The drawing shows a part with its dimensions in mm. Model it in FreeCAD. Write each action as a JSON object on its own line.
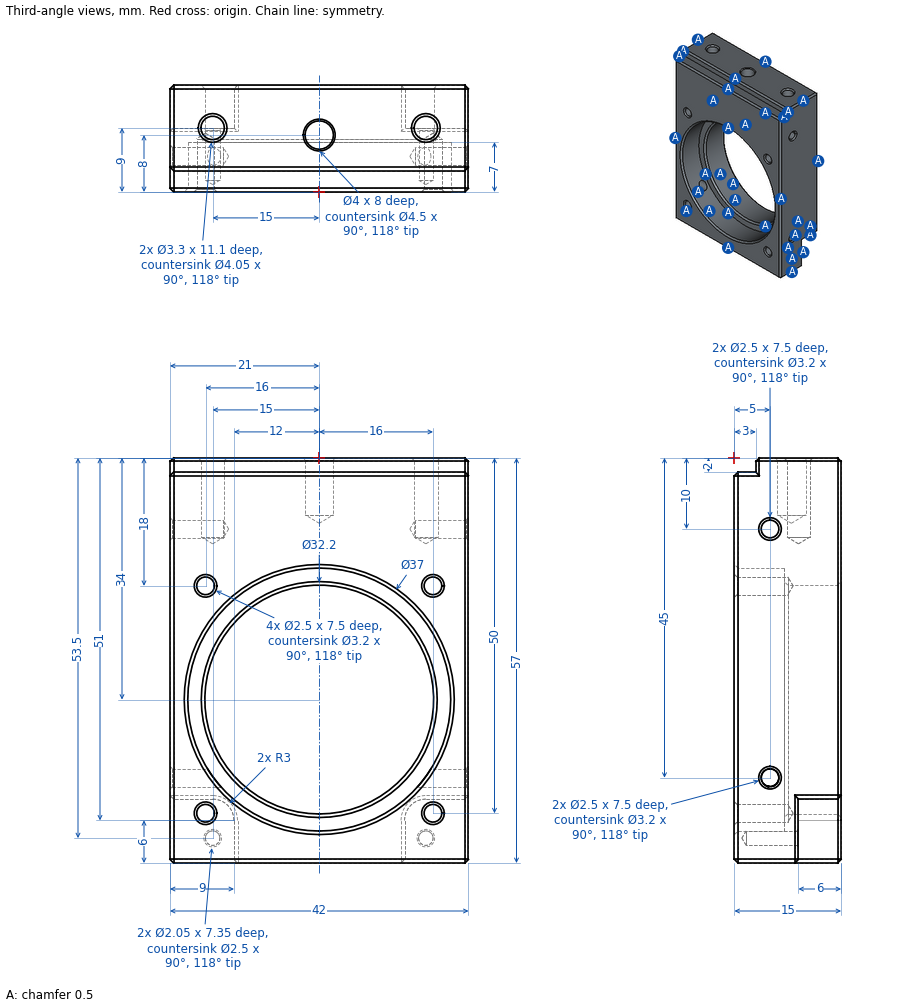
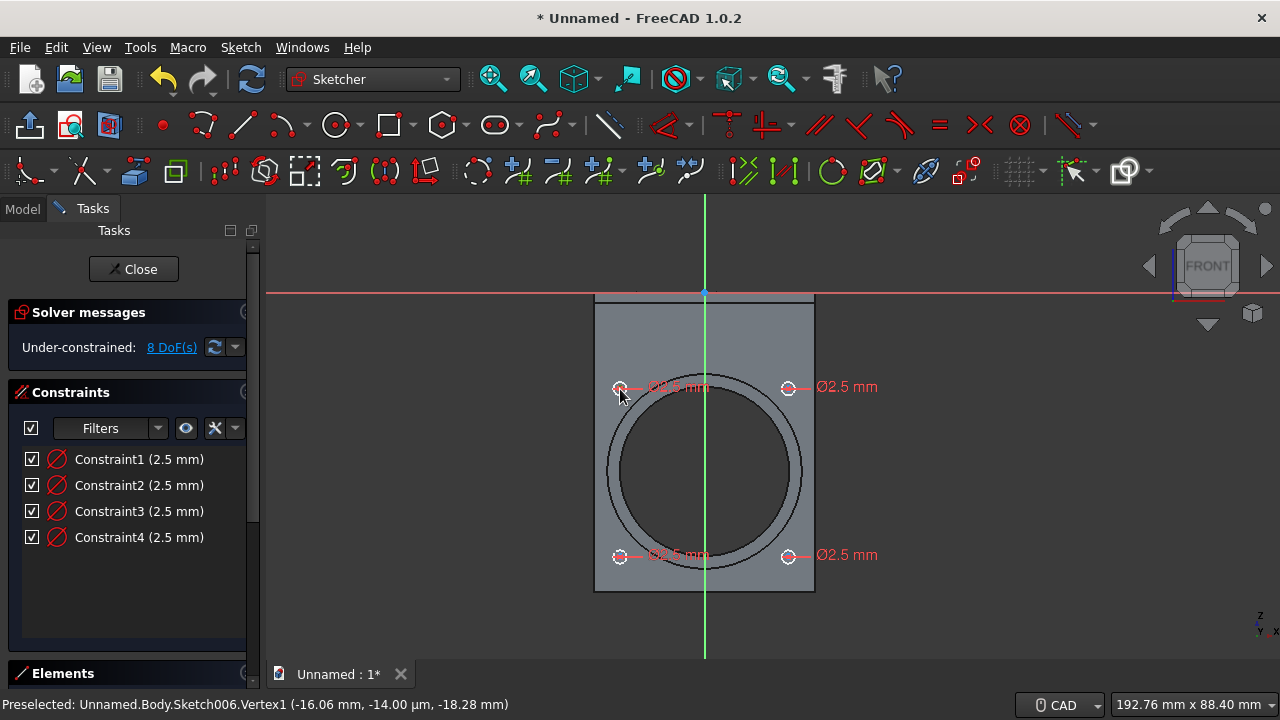
{"action": "left_click", "coordinate": [788, 389]}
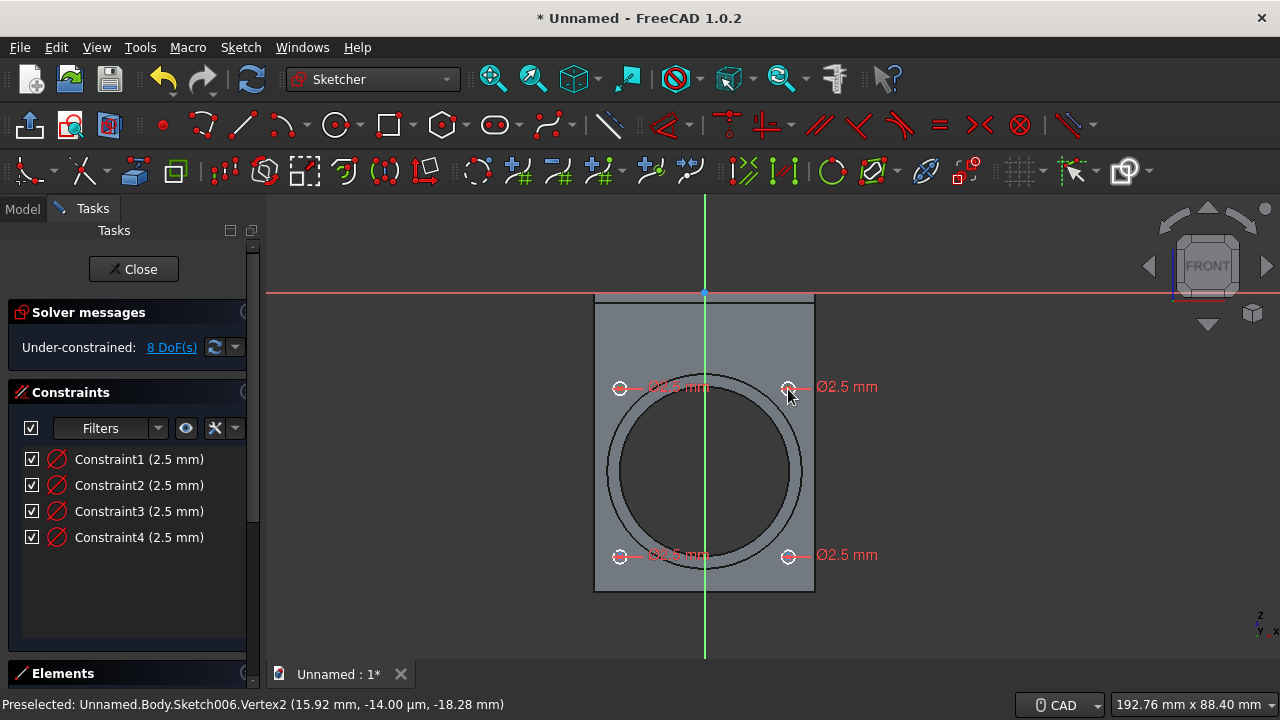
{"action": "left_click", "coordinate": [705, 602]}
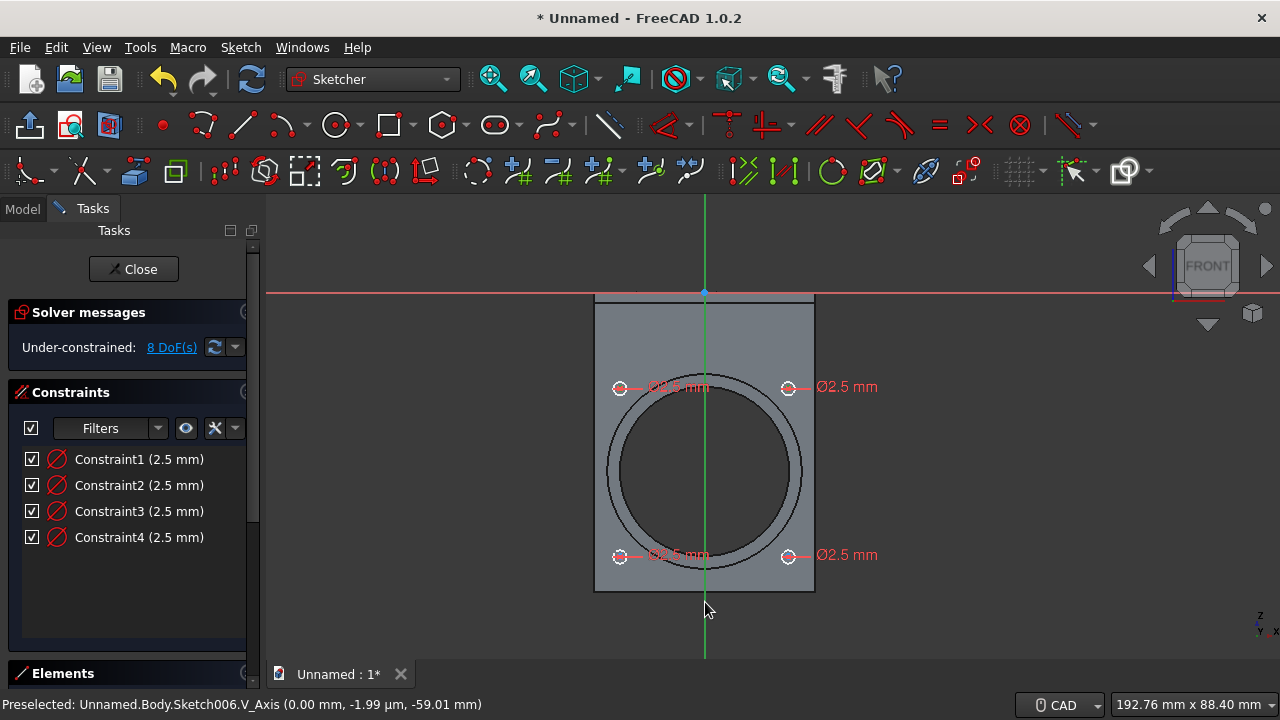
{"action": "key", "text": "s"}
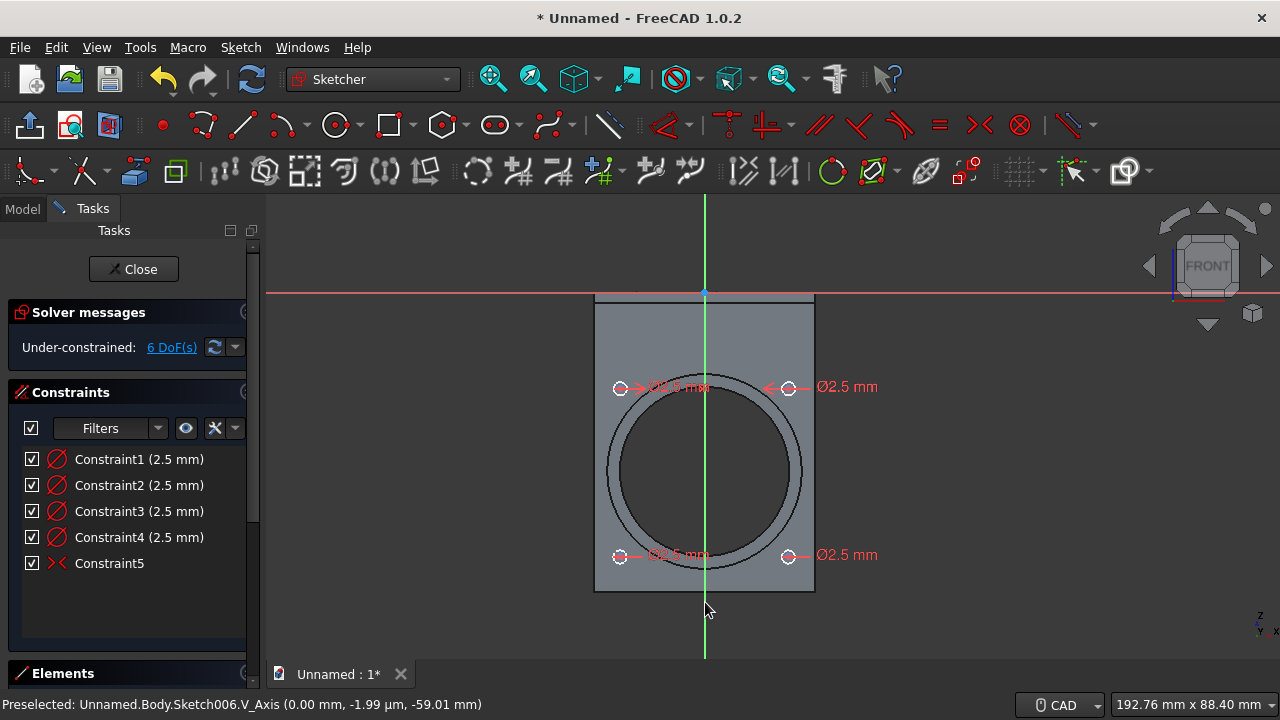
{"action": "left_click", "coordinate": [788, 557]}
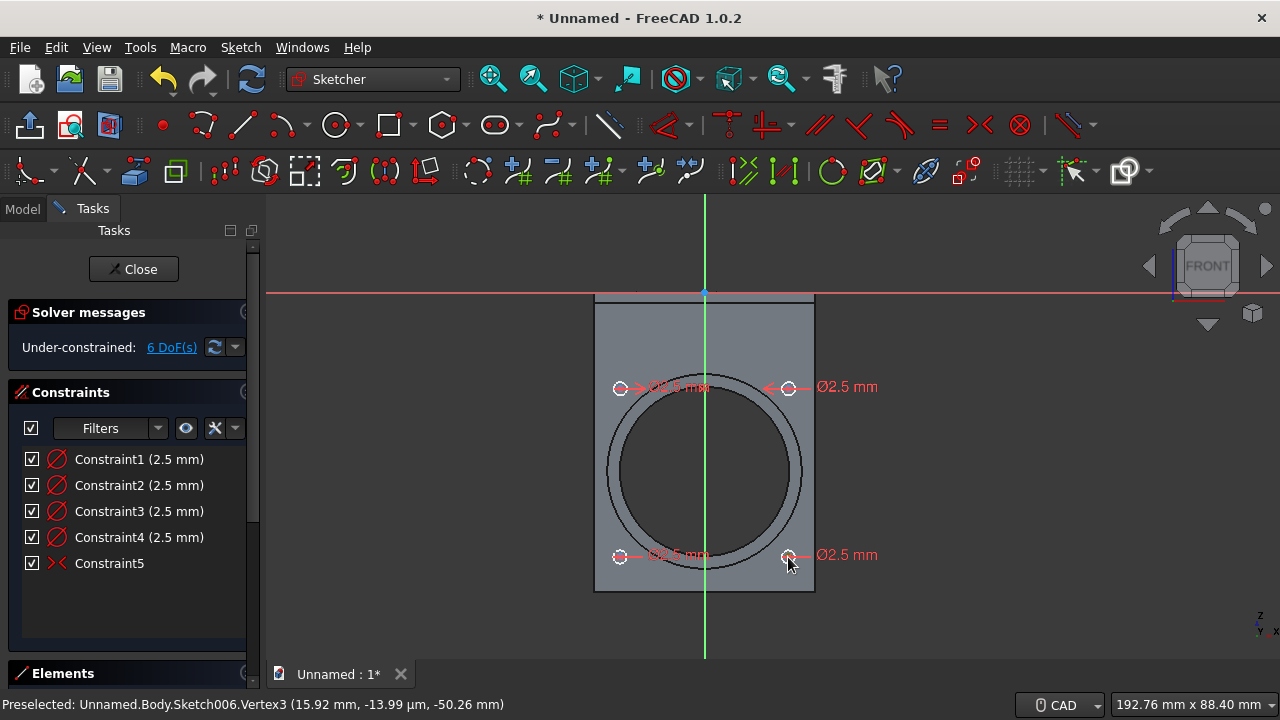
{"action": "left_click", "coordinate": [620, 557]}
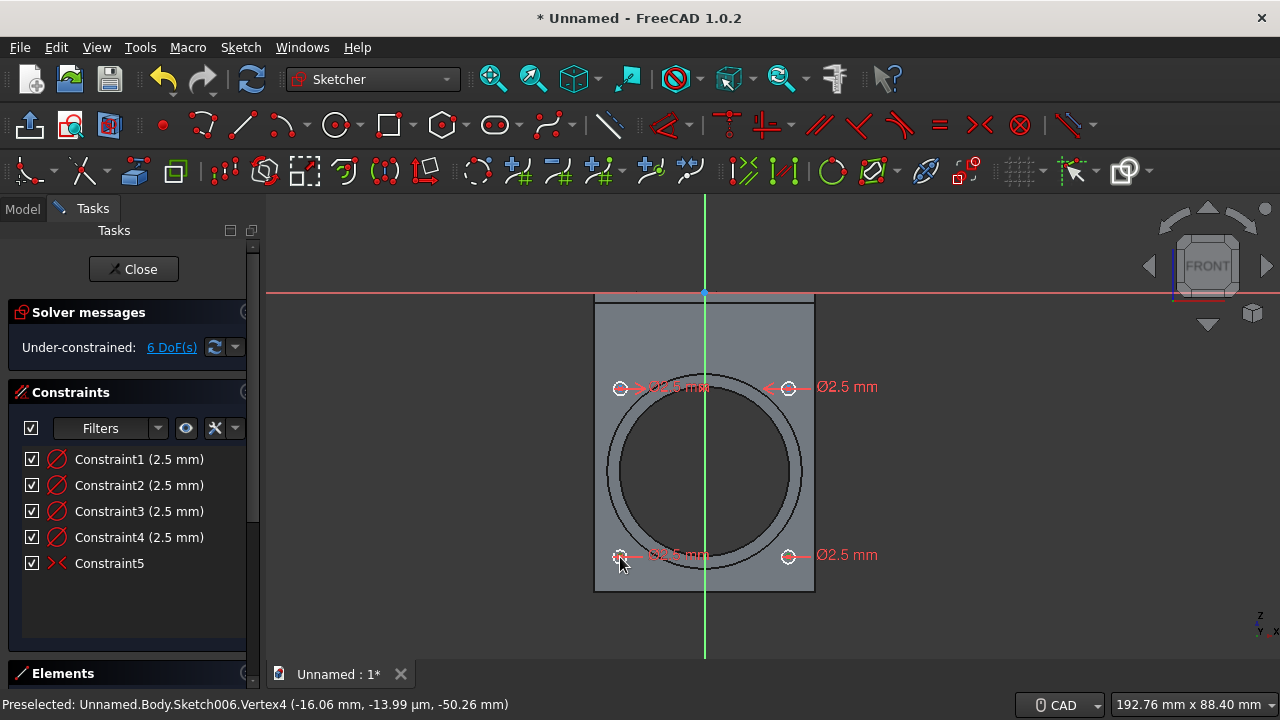
{"action": "left_click", "coordinate": [705, 602]}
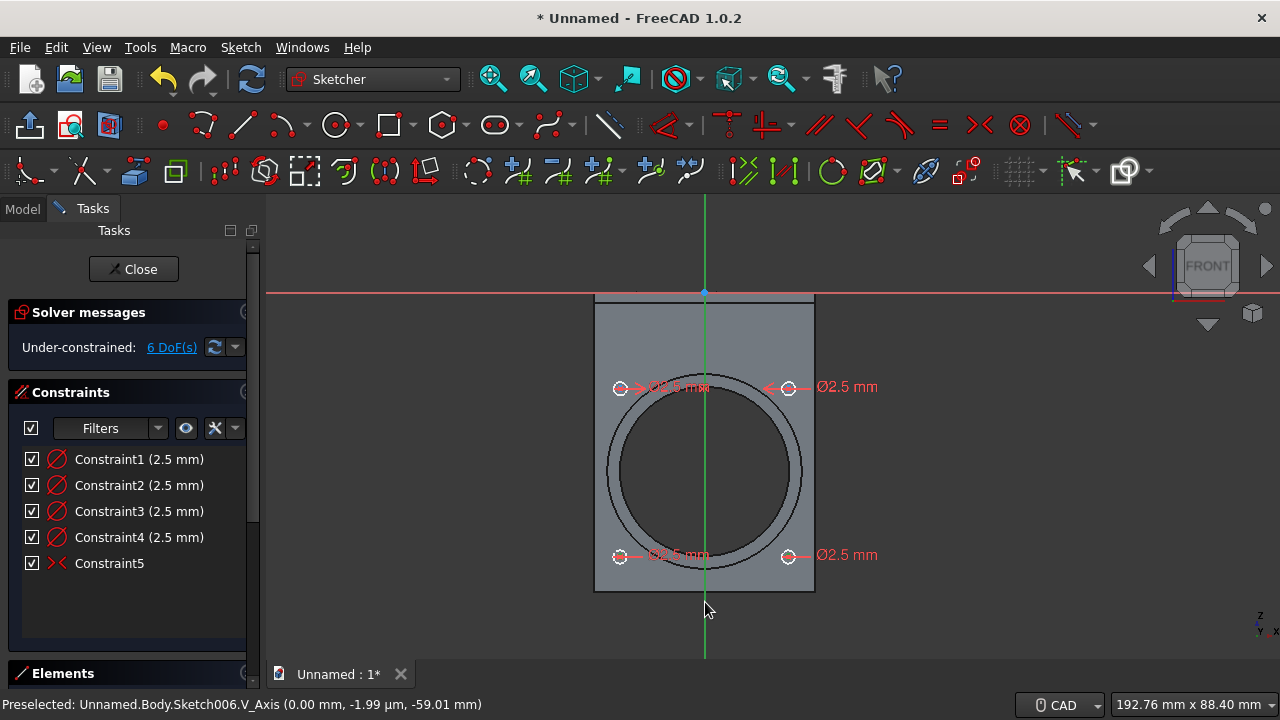
{"action": "left_click", "coordinate": [980, 126]}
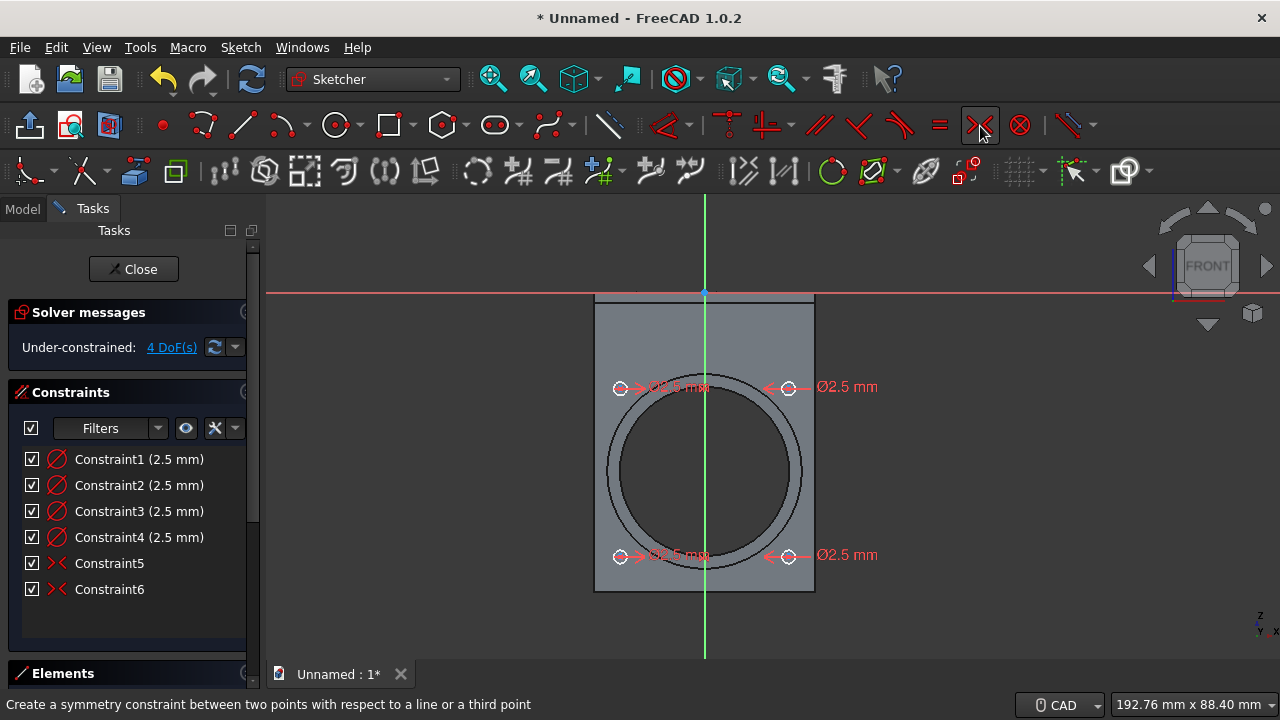
{"action": "key", "text": "d"}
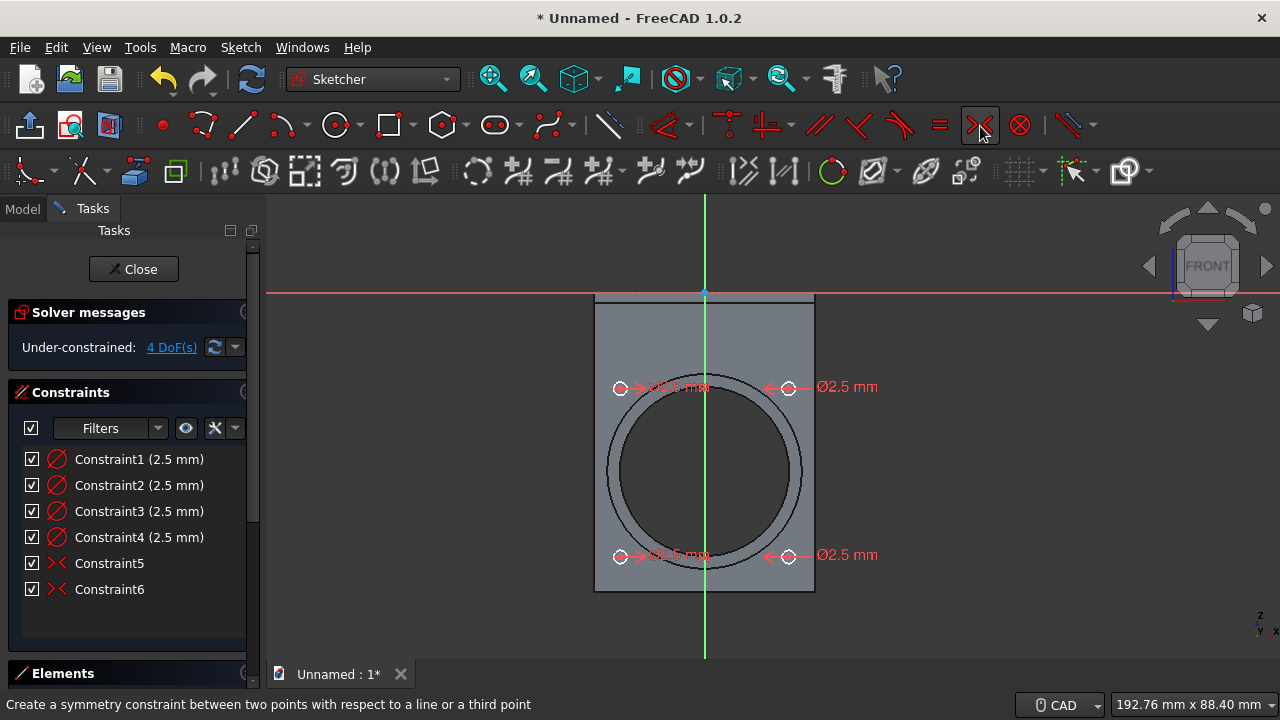
{"action": "left_click", "coordinate": [620, 389]}
{"action": "left_click", "coordinate": [662, 259]}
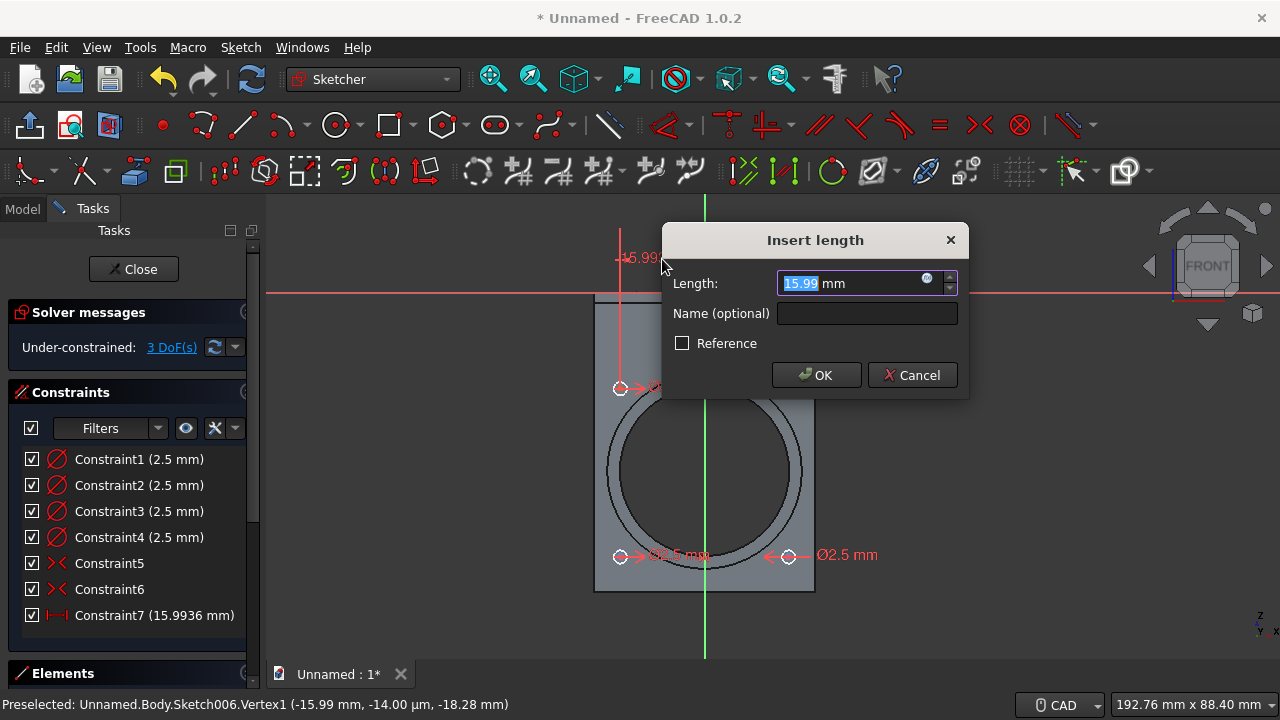
{"action": "type", "text": "16"}
{"action": "key", "text": "Return"}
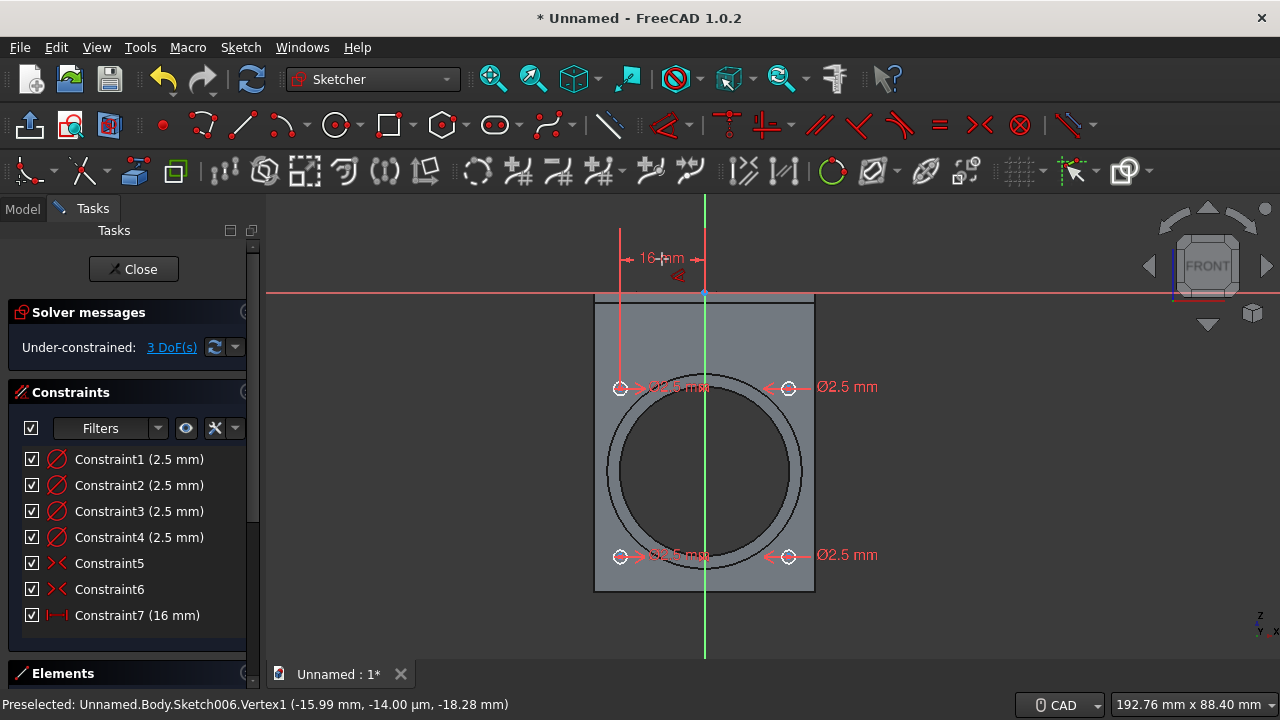
{"action": "left_click", "coordinate": [620, 389]}
{"action": "left_click", "coordinate": [586, 341]}